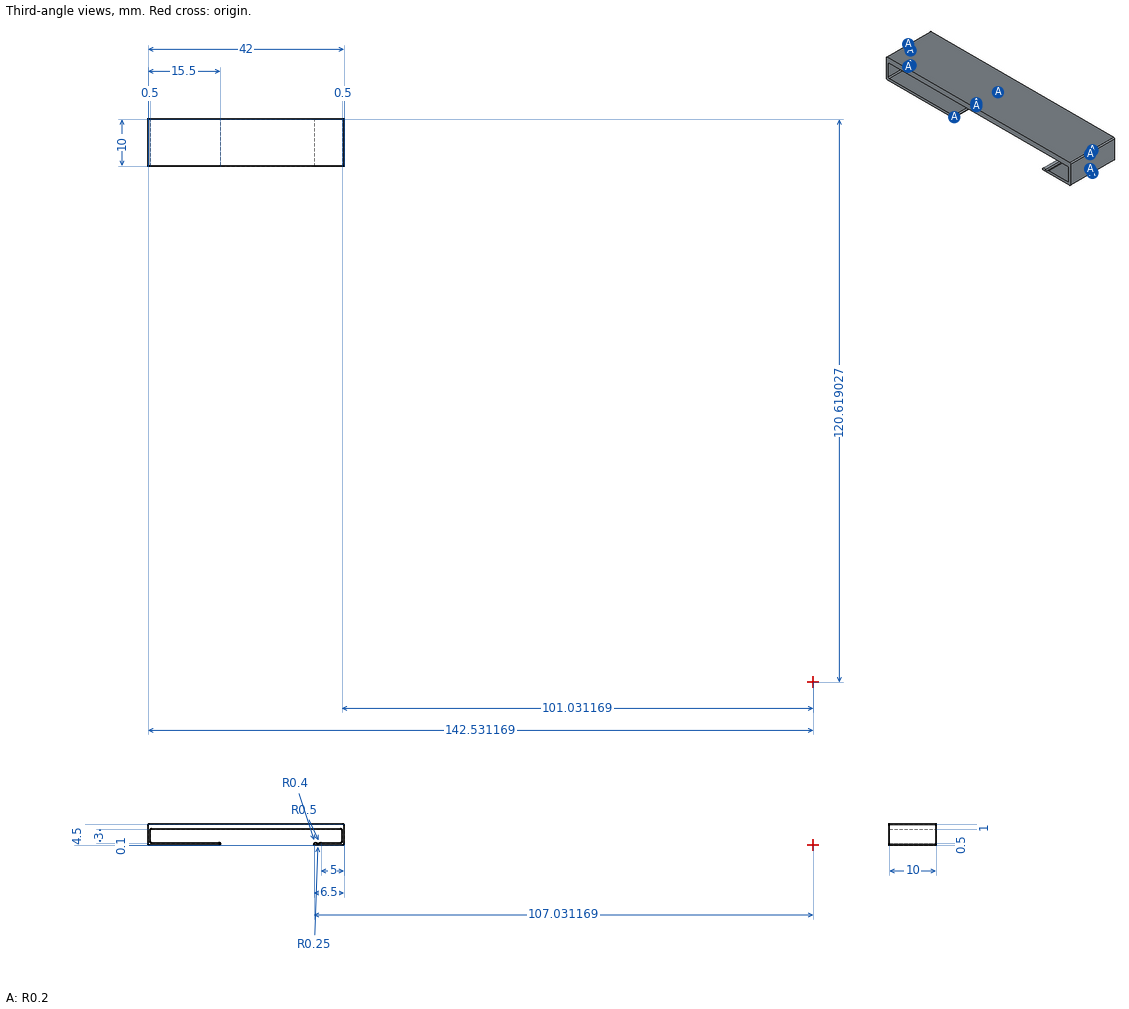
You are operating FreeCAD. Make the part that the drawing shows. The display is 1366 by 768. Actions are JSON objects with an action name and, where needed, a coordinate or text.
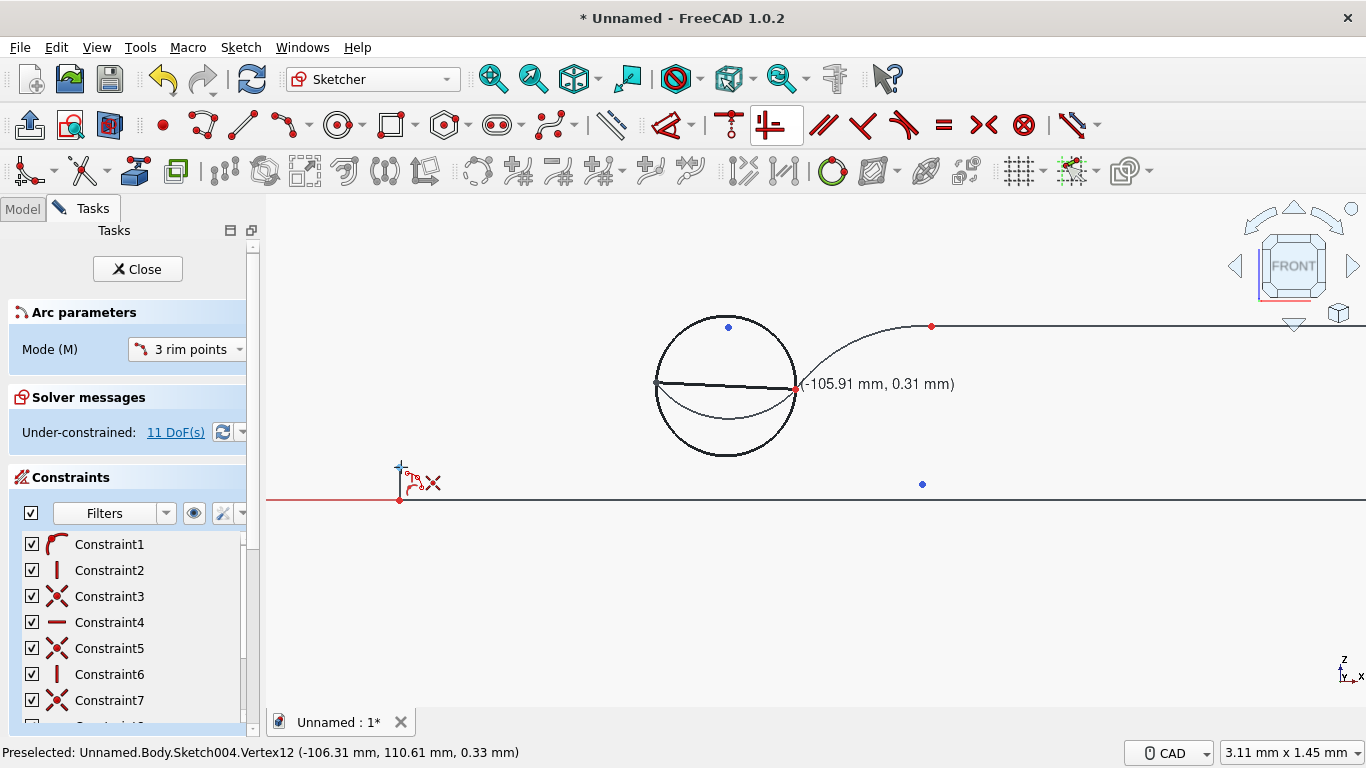
{"action": "left_click", "coordinate": [400, 467]}
{"action": "left_click", "coordinate": [498, 330]}
{"action": "key", "text": "Escape"}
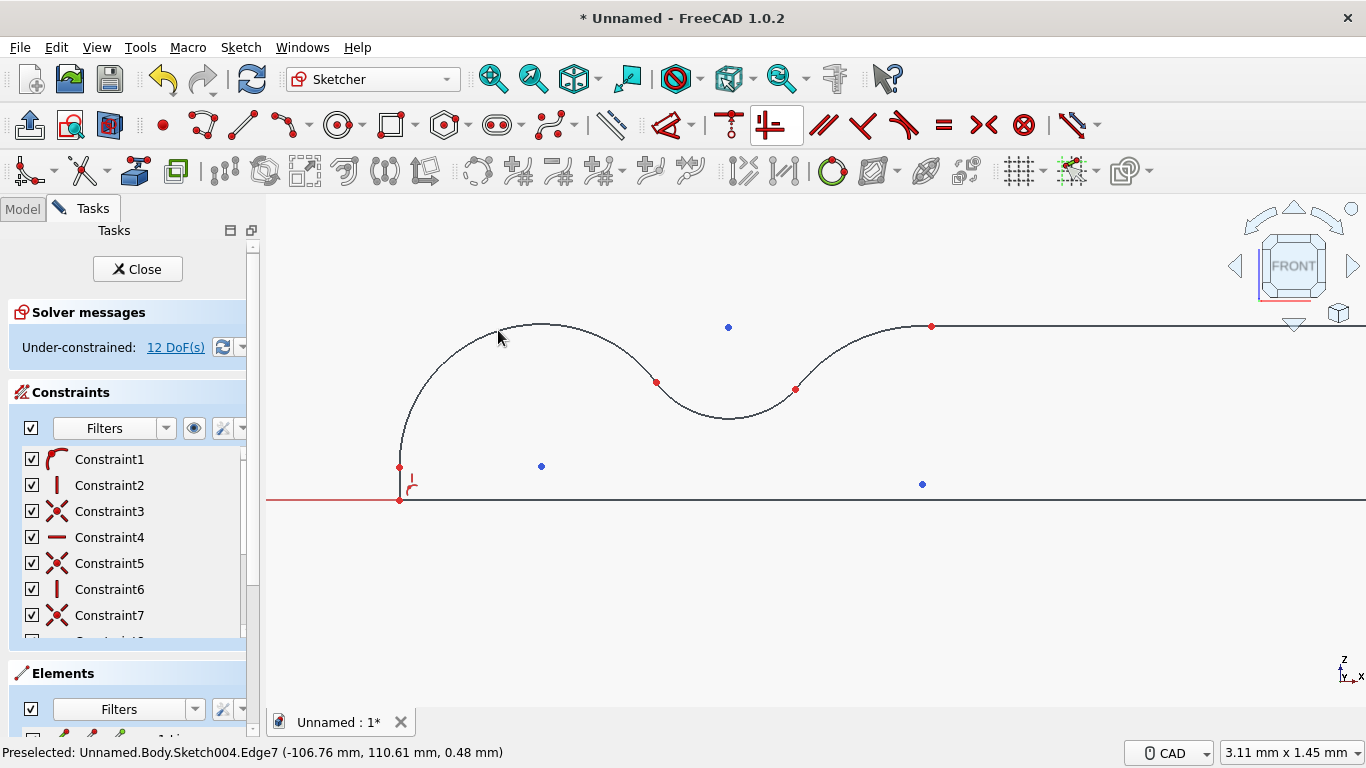
{"action": "scroll", "coordinate": [400, 477], "scroll_direction": "up", "scroll_amount": 2}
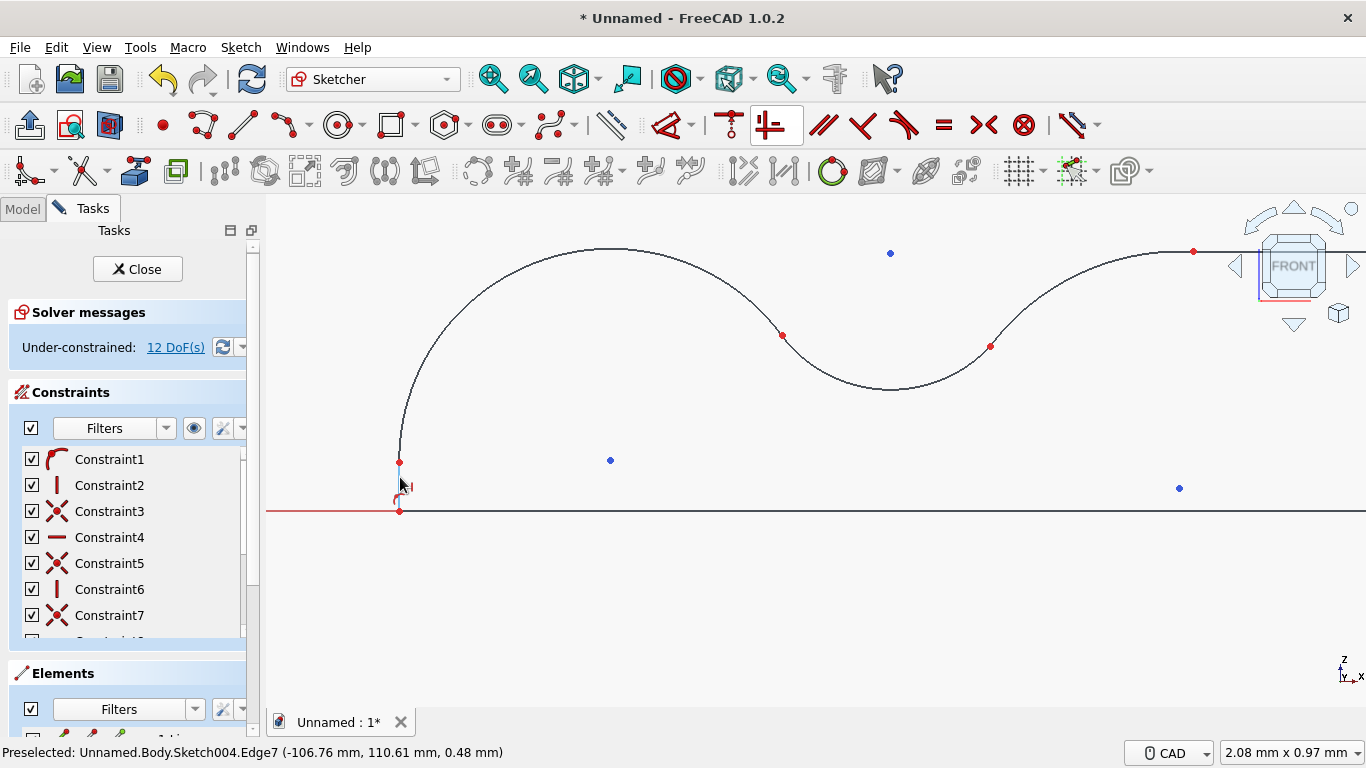
{"action": "left_click", "coordinate": [399, 477]}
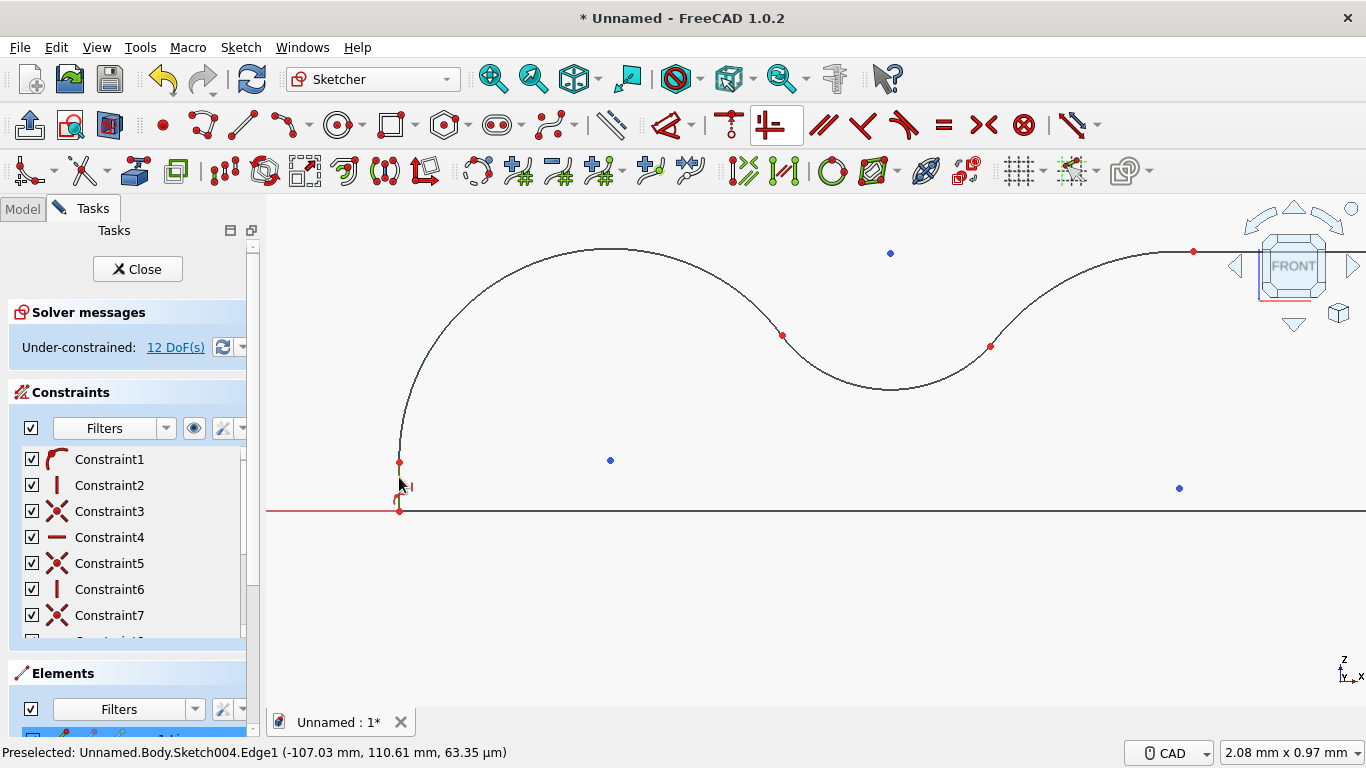
{"action": "scroll", "coordinate": [401, 468], "scroll_direction": "down", "scroll_amount": 8}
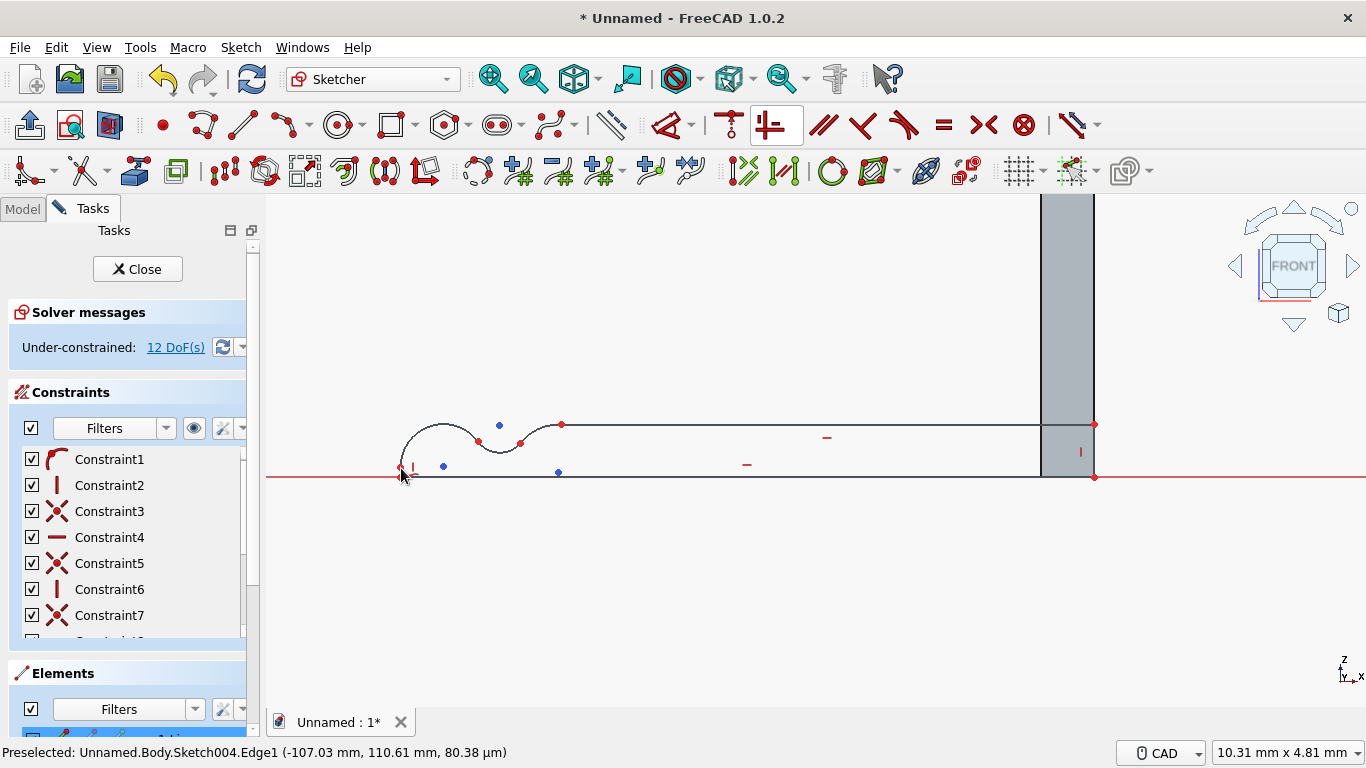
{"action": "left_click", "coordinate": [451, 425]}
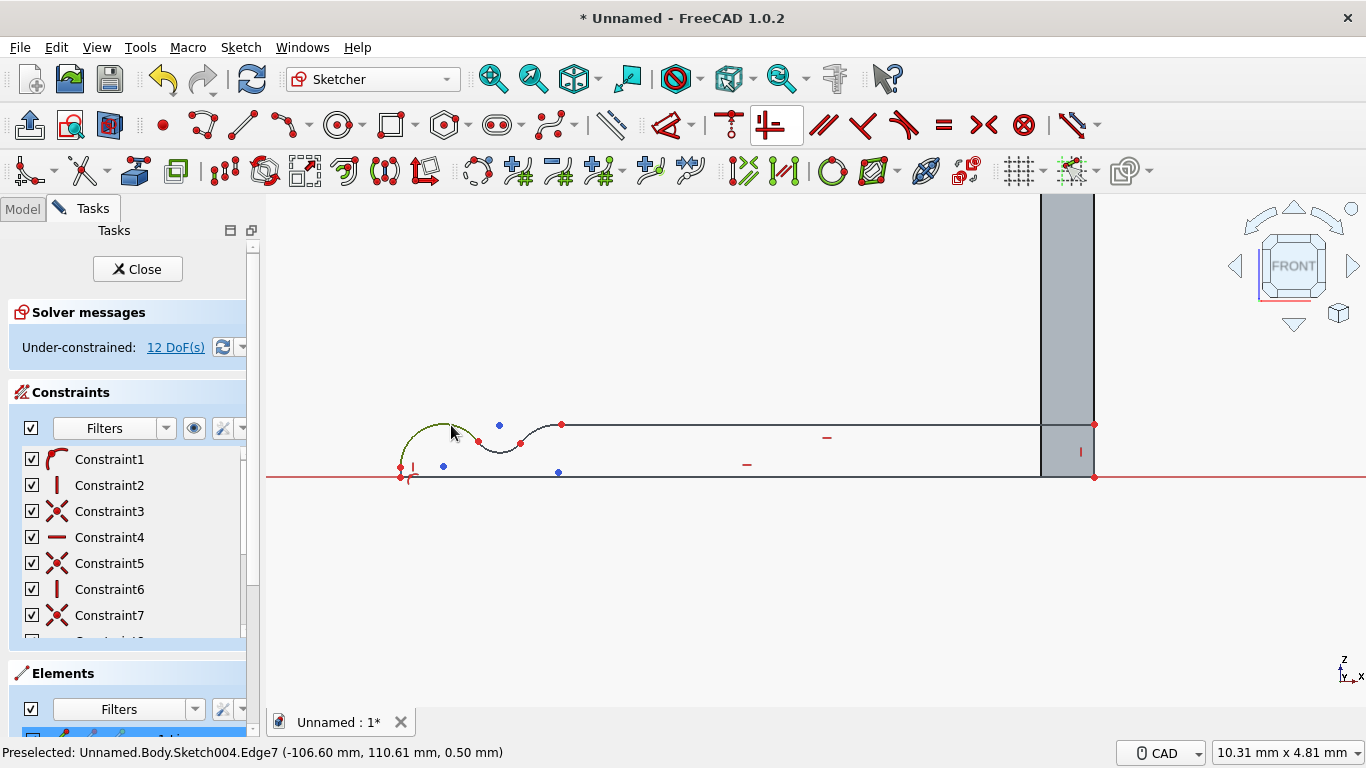
{"action": "left_click", "coordinate": [904, 126]}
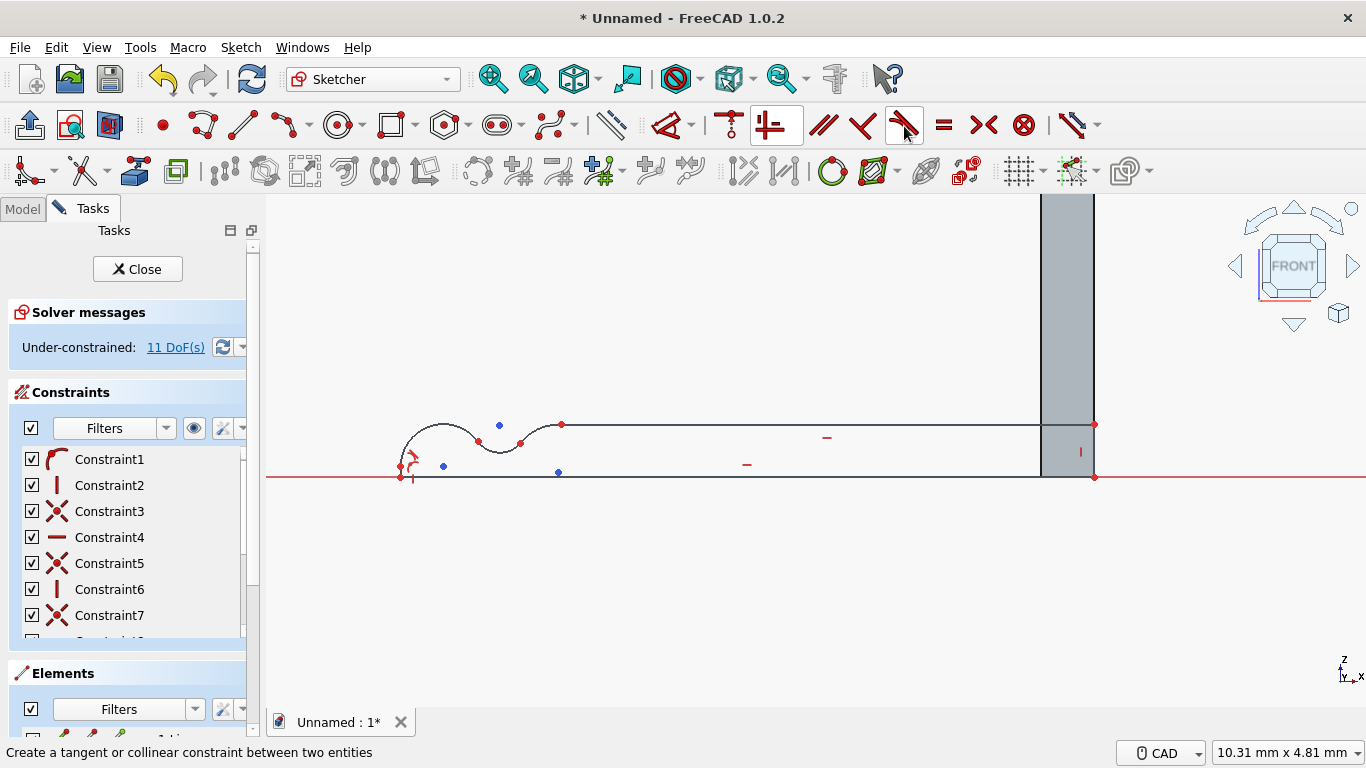
{"action": "left_click", "coordinate": [934, 425]}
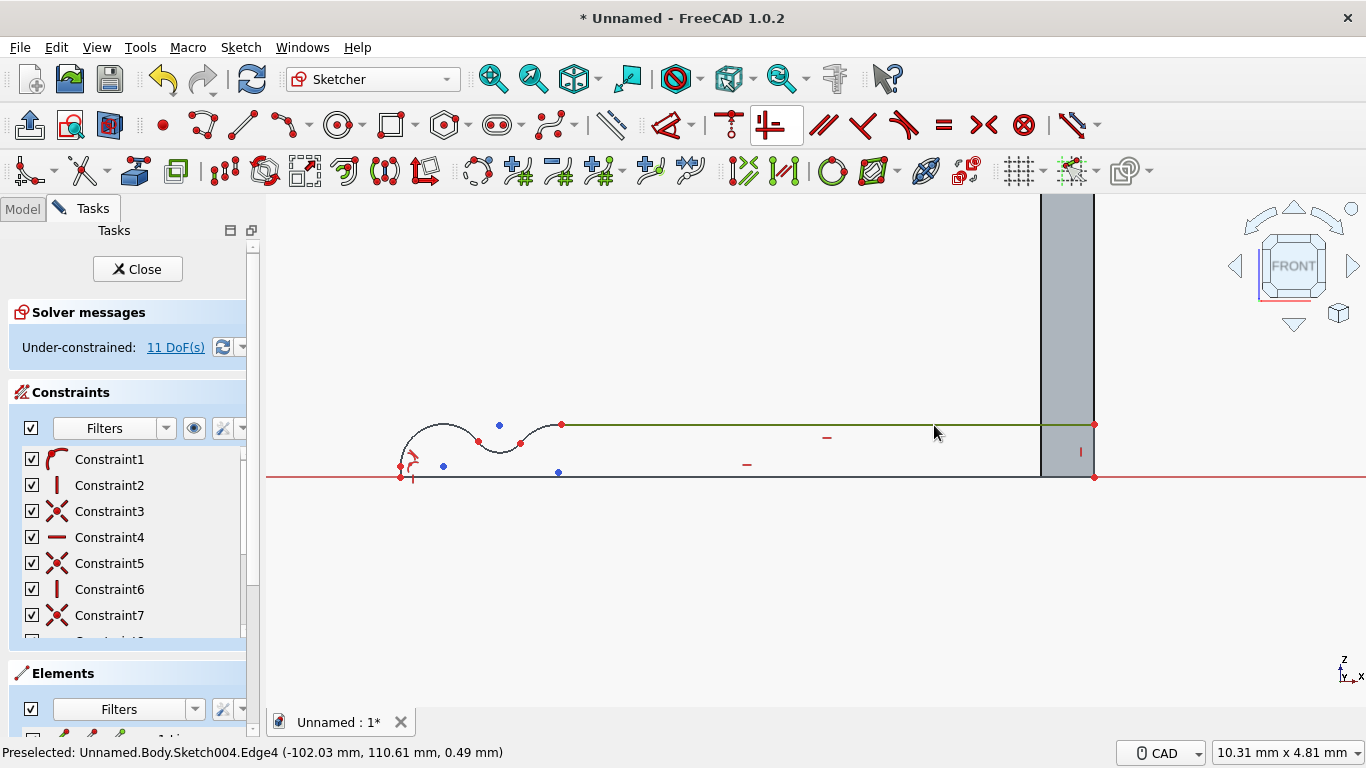
{"action": "left_click", "coordinate": [547, 426]}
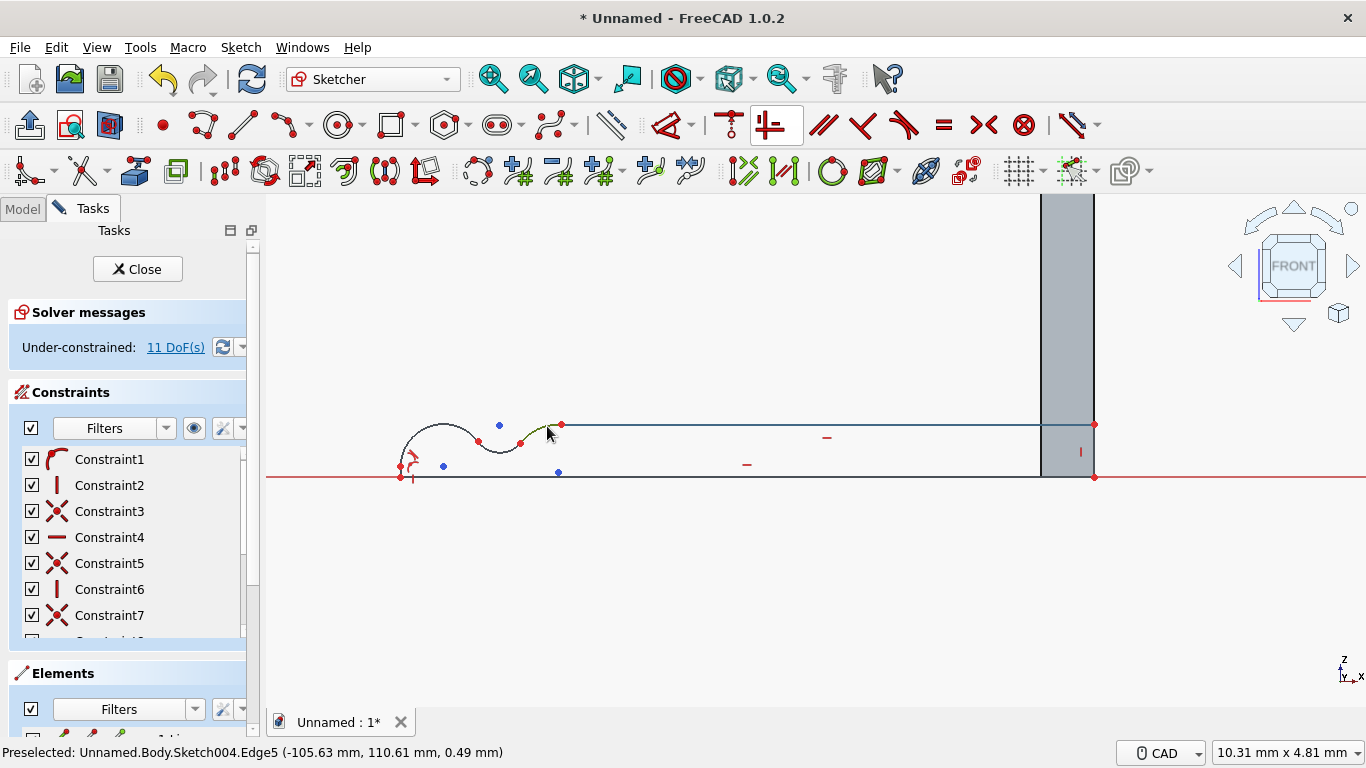
{"action": "left_click", "coordinate": [904, 126]}